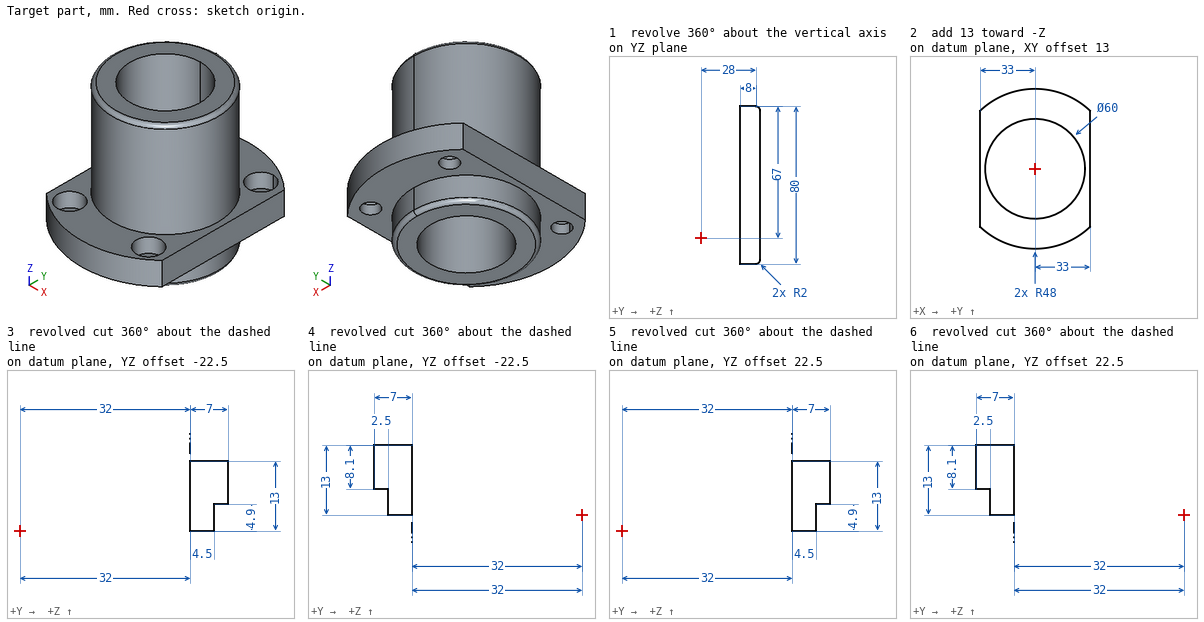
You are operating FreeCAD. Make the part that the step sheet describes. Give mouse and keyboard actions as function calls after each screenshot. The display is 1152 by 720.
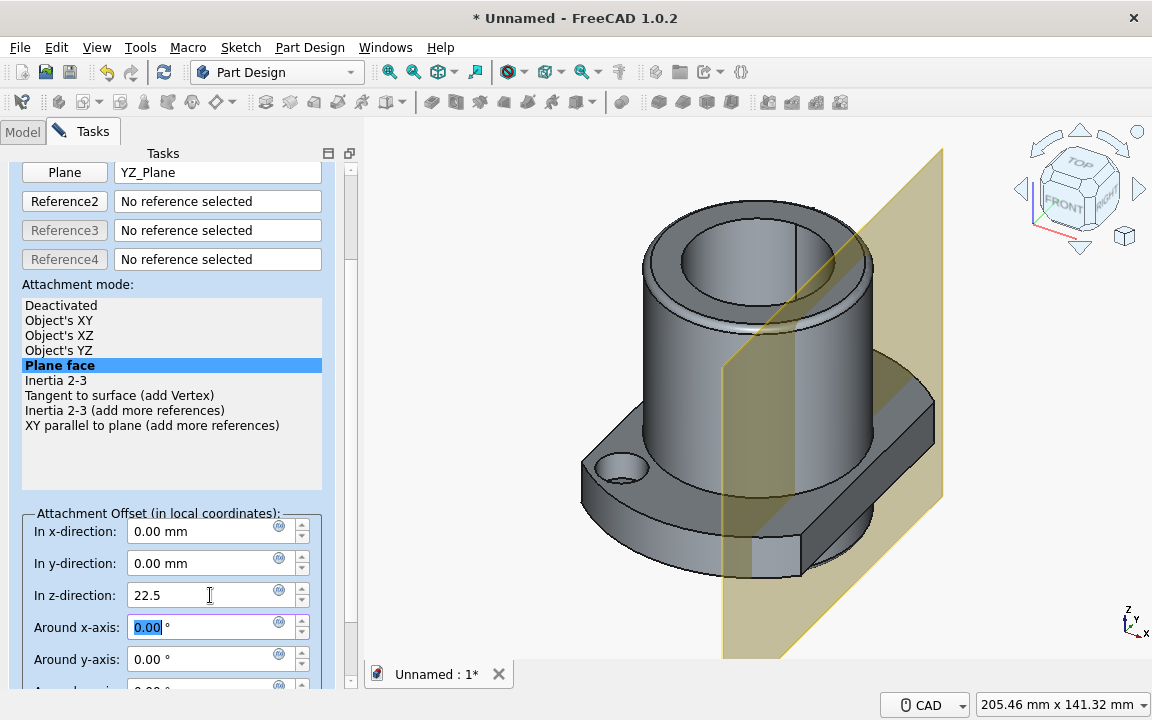
scroll(351, 426, up, 3)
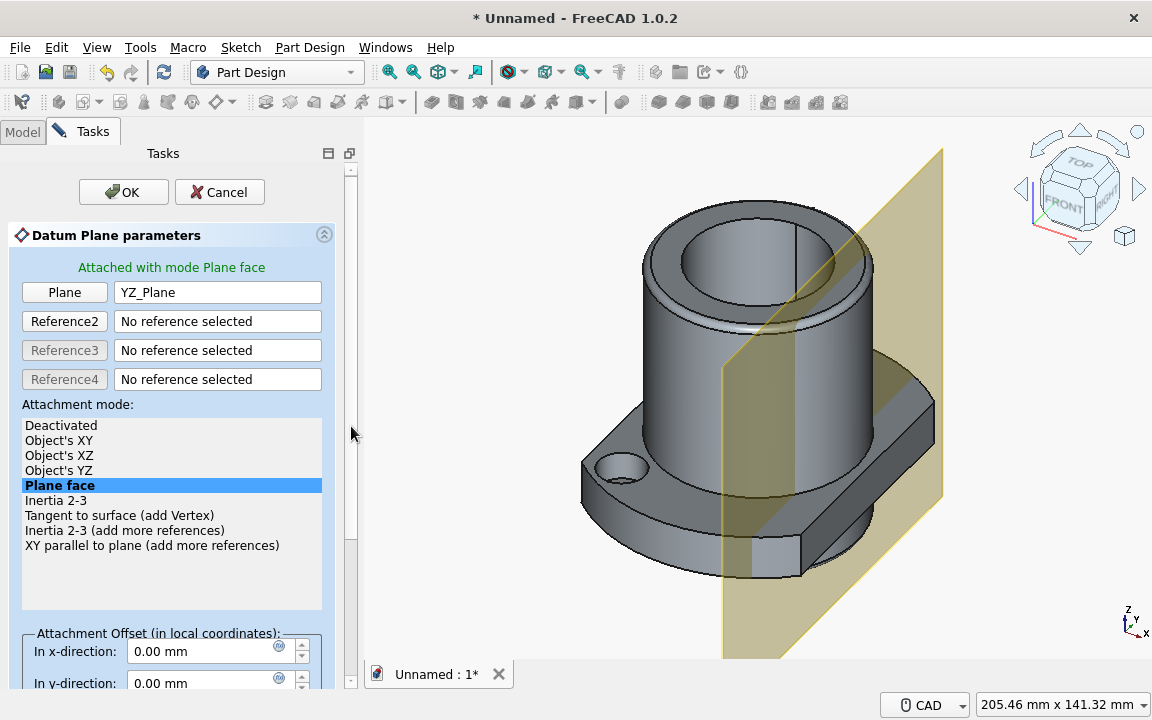
click(124, 192)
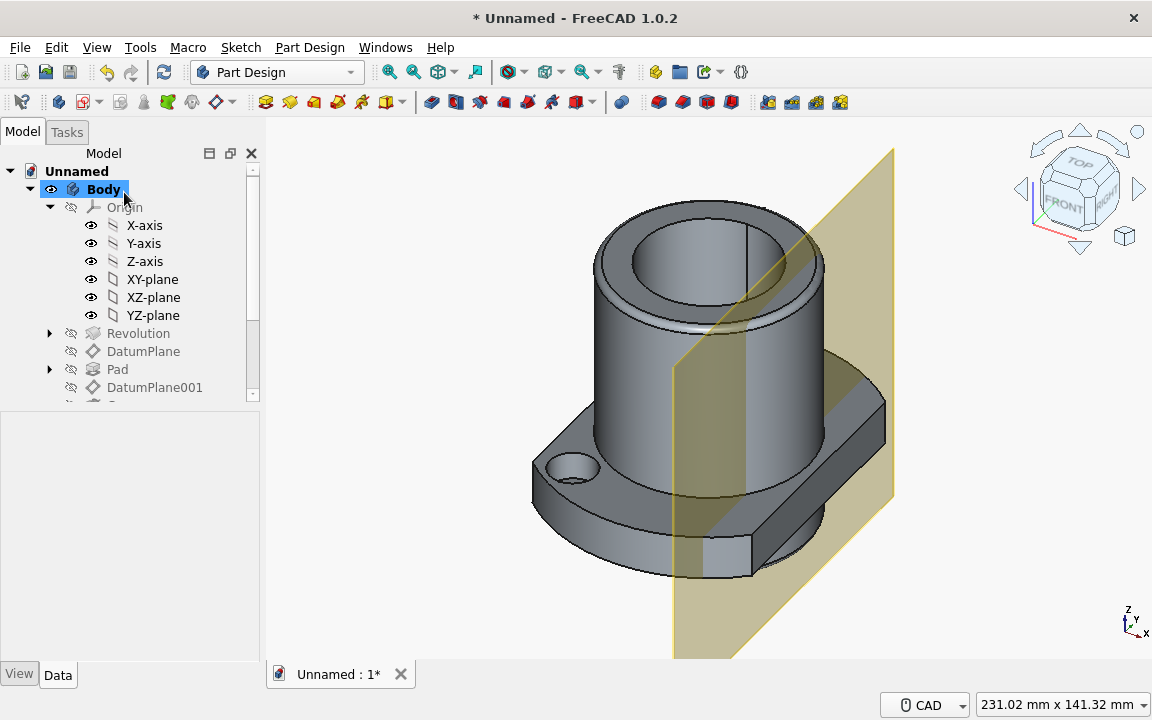
scroll(100, 275, down, 3)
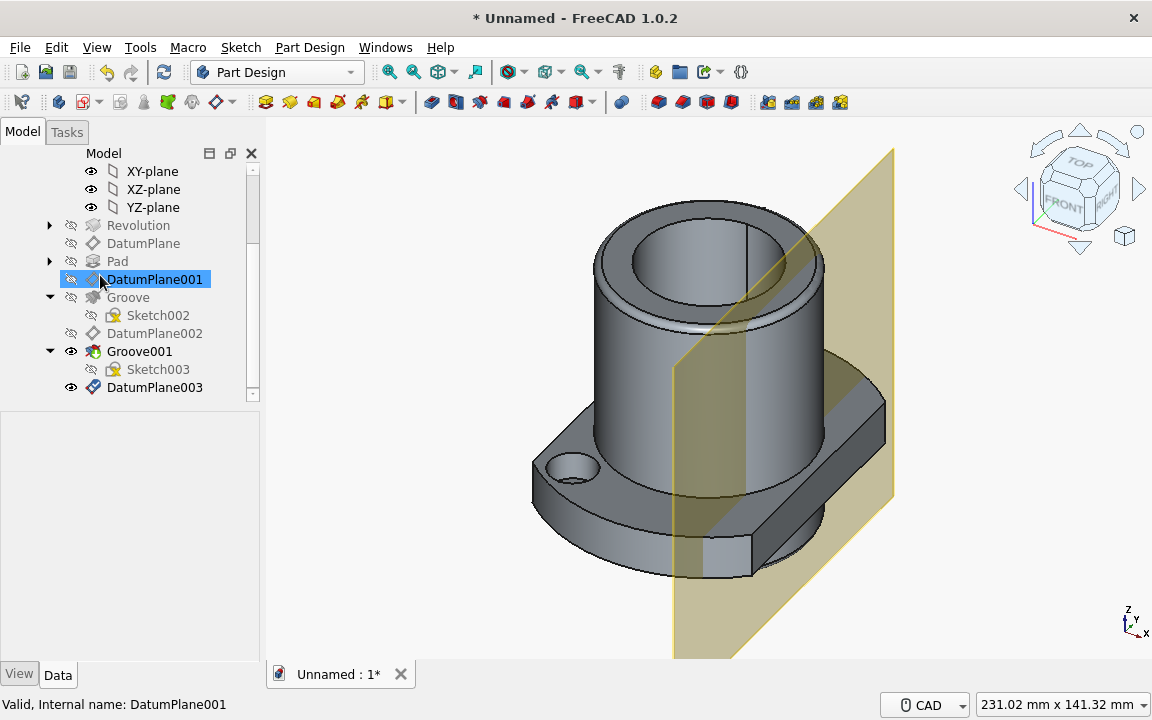
click(116, 387)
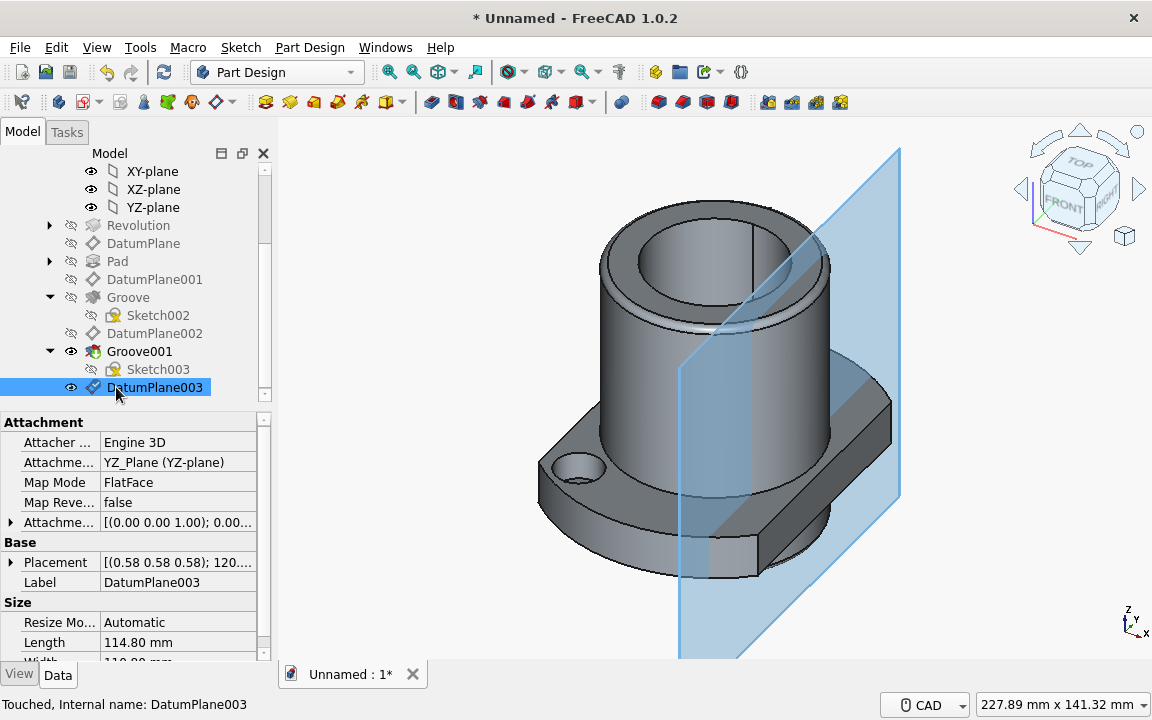
click(84, 102)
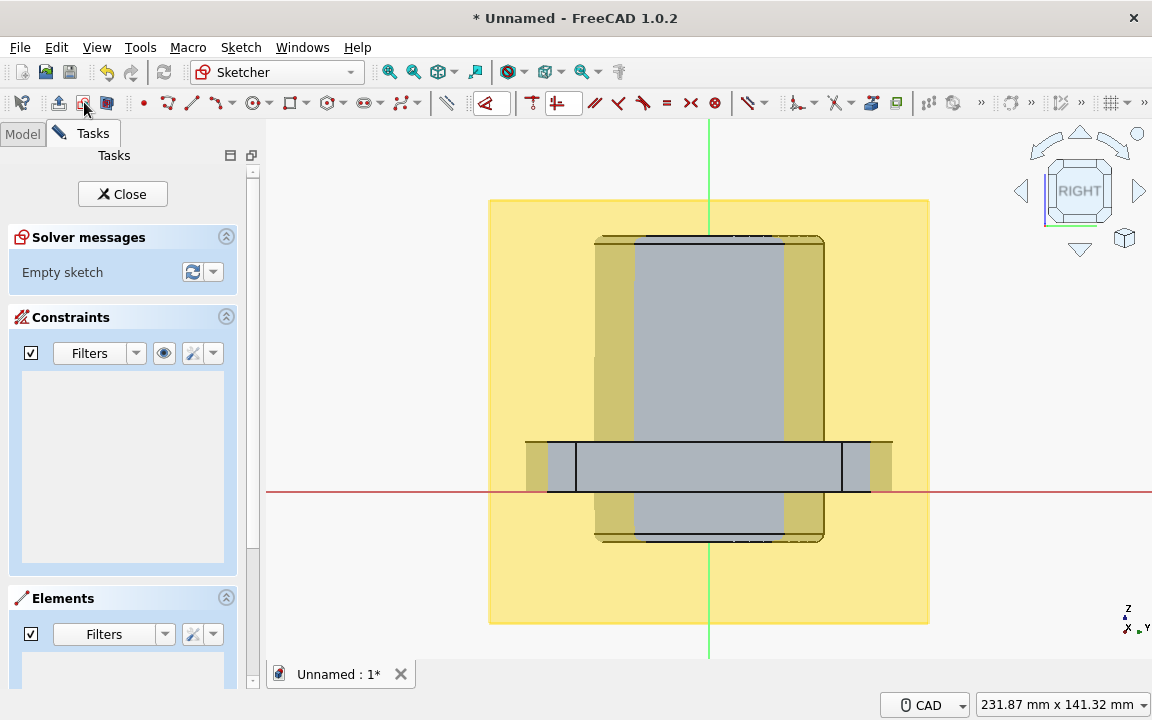
click(108, 104)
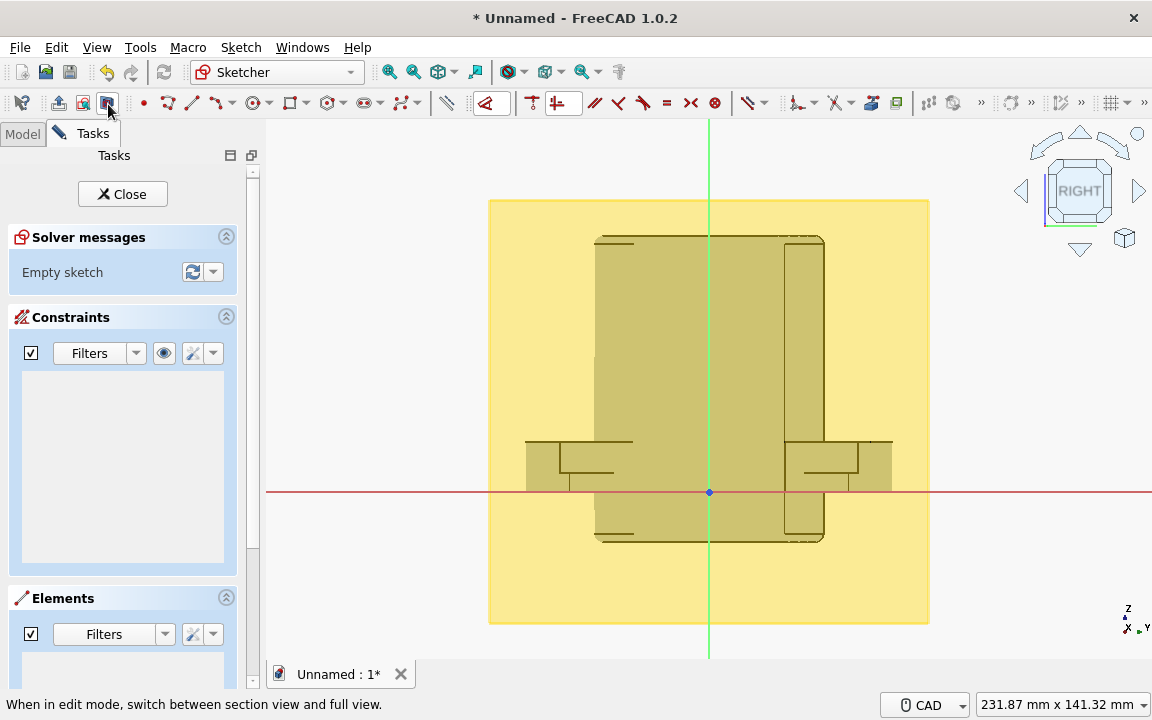
scroll(845, 487, up, 6)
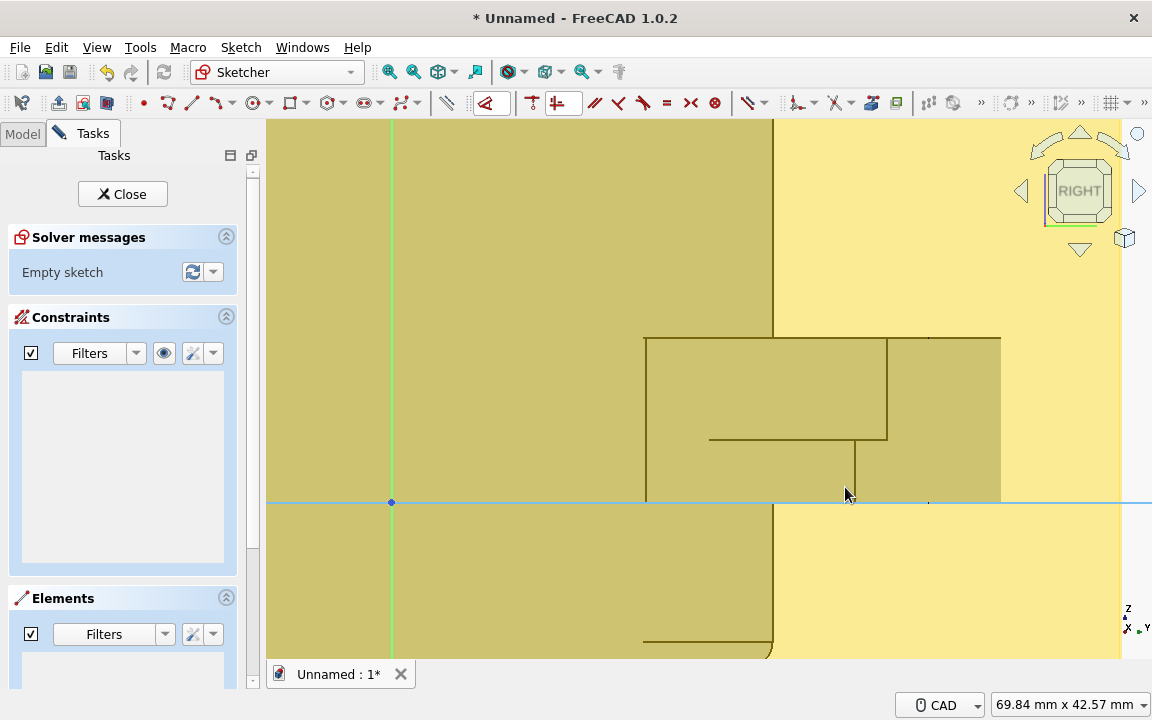
click(168, 104)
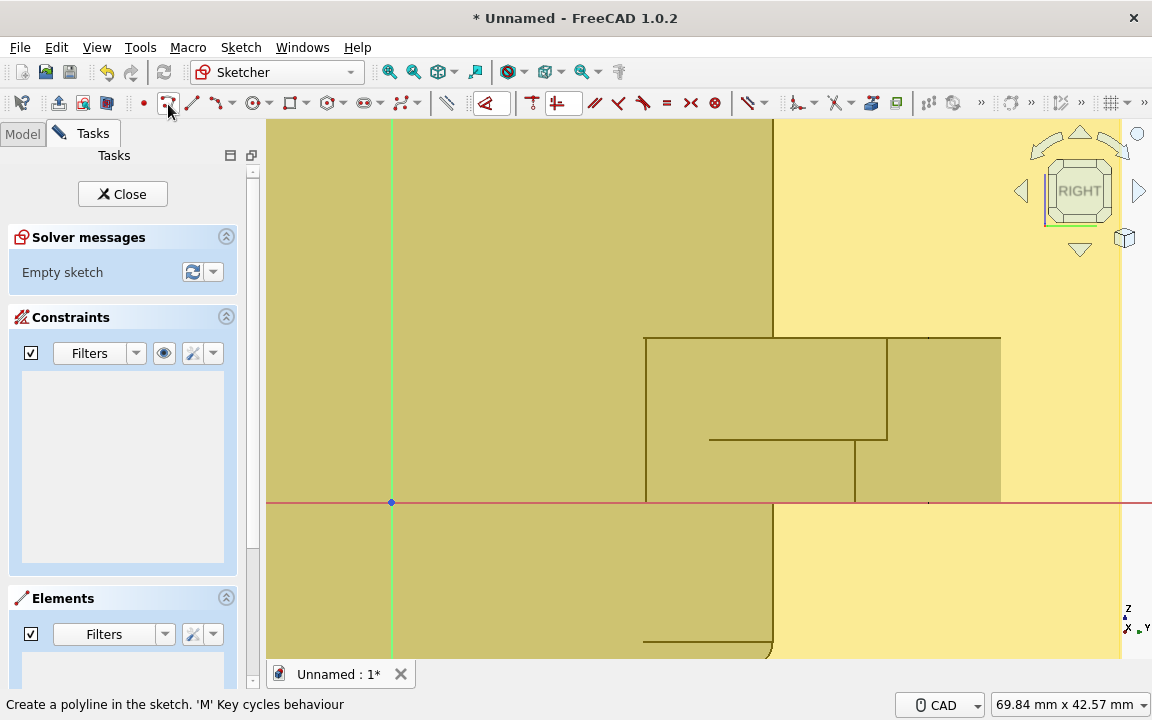
click(798, 503)
click(855, 494)
click(855, 440)
click(887, 440)
click(887, 338)
click(798, 338)
click(798, 503)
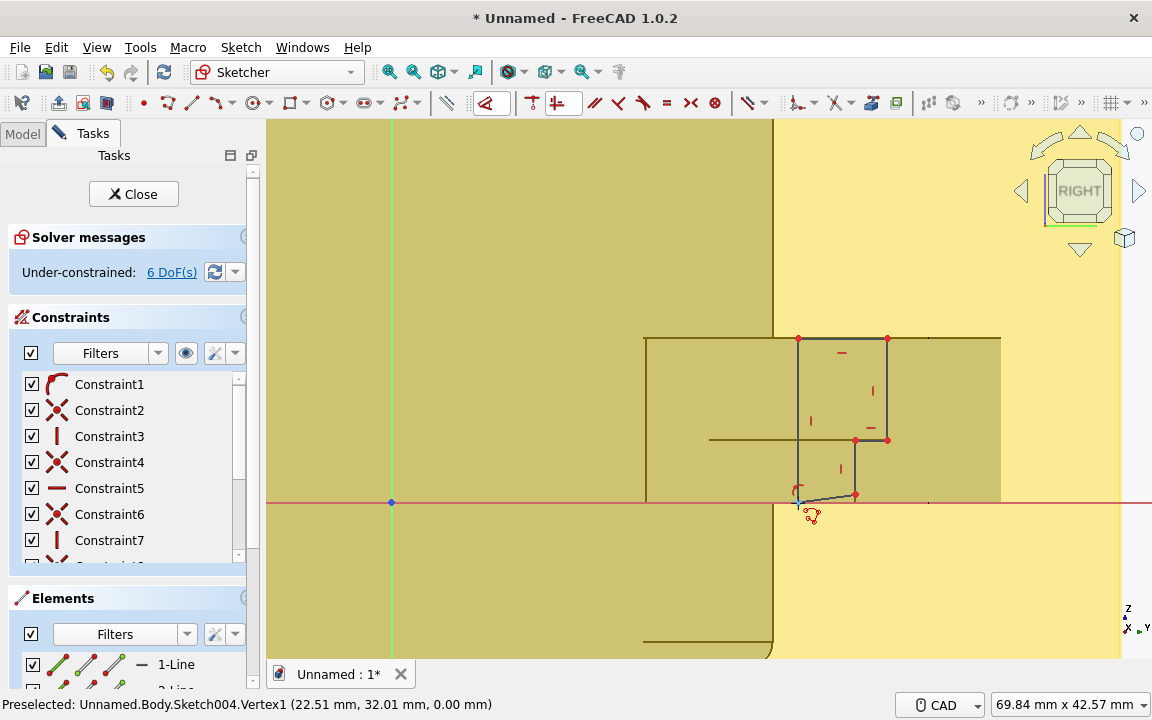
click(192, 104)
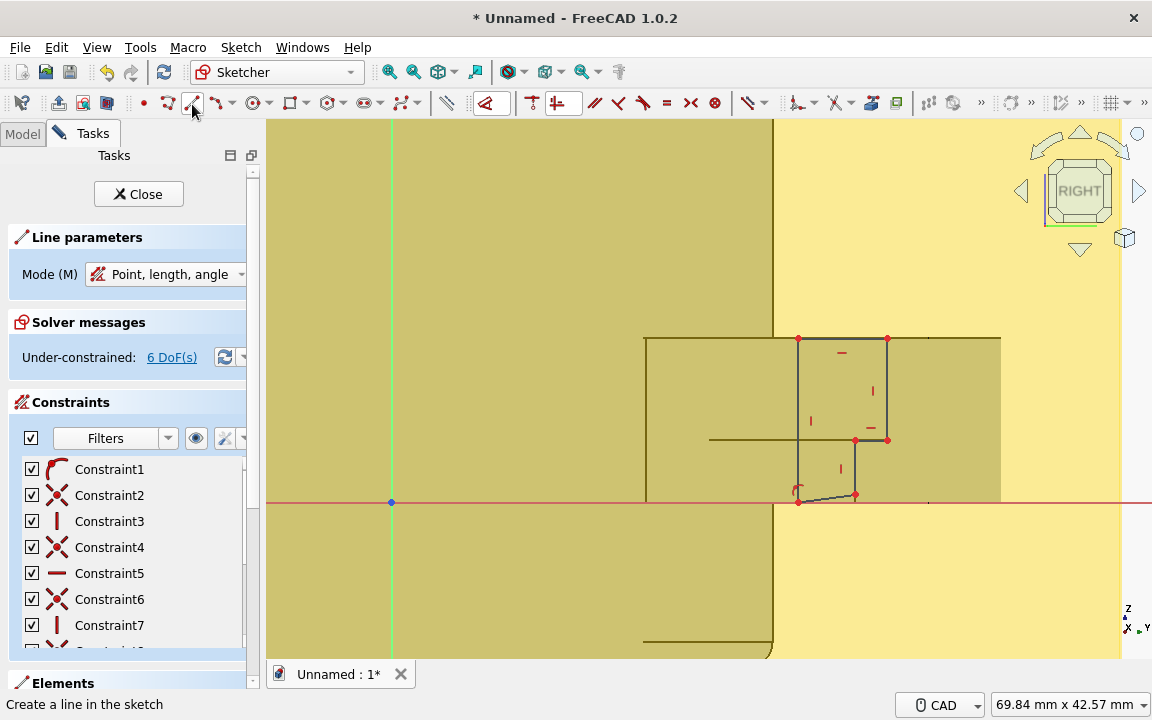
click(798, 321)
click(798, 272)
key(Escape)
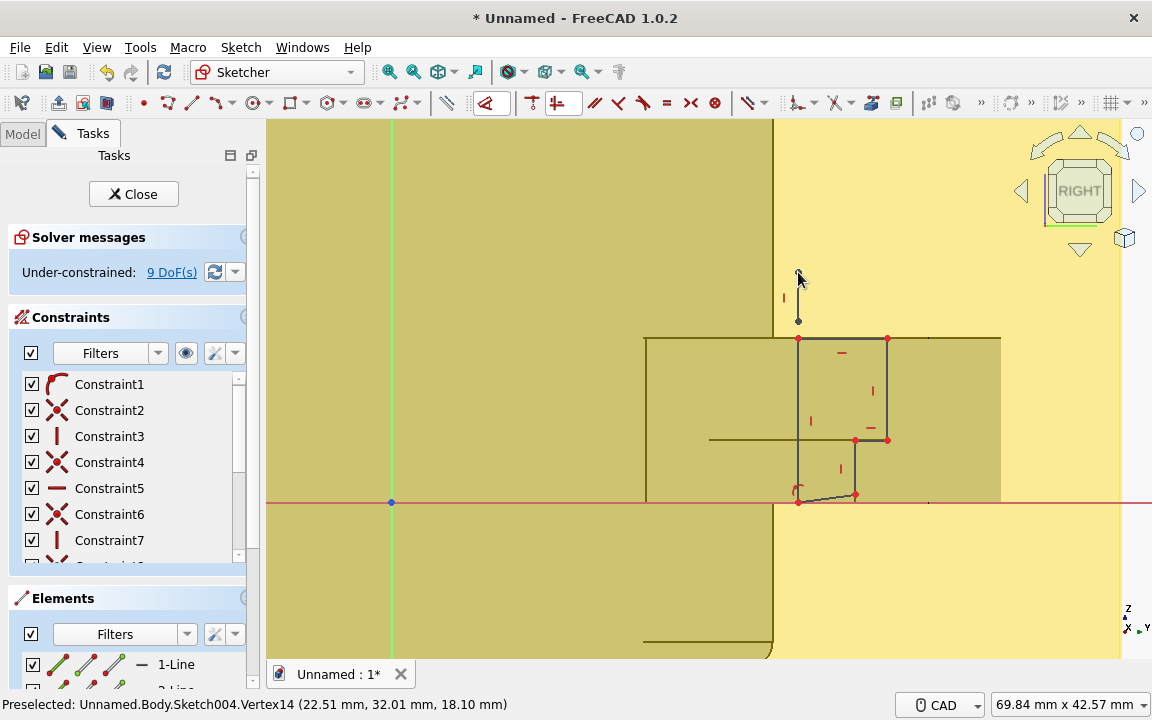
click(798, 307)